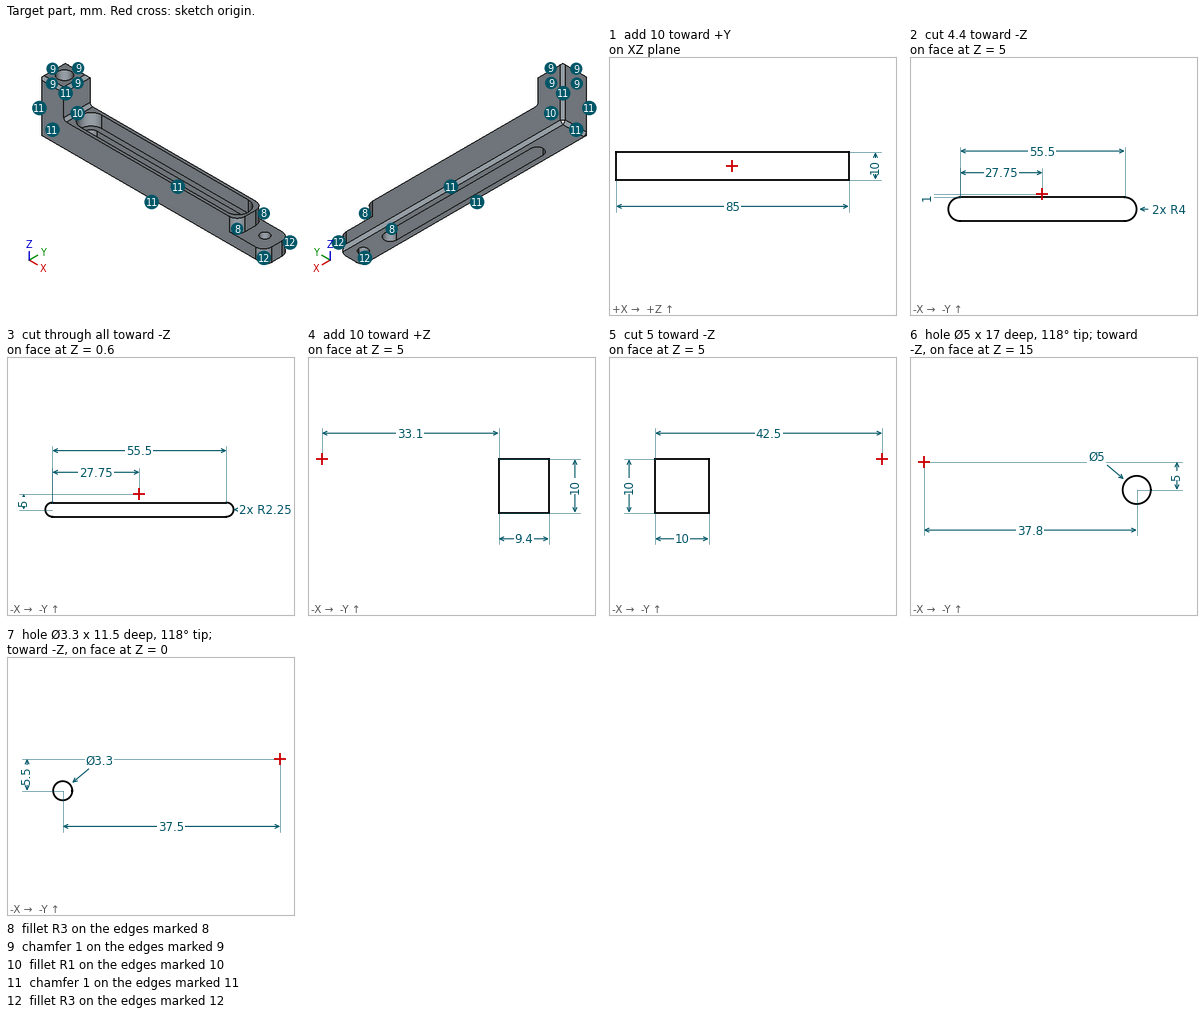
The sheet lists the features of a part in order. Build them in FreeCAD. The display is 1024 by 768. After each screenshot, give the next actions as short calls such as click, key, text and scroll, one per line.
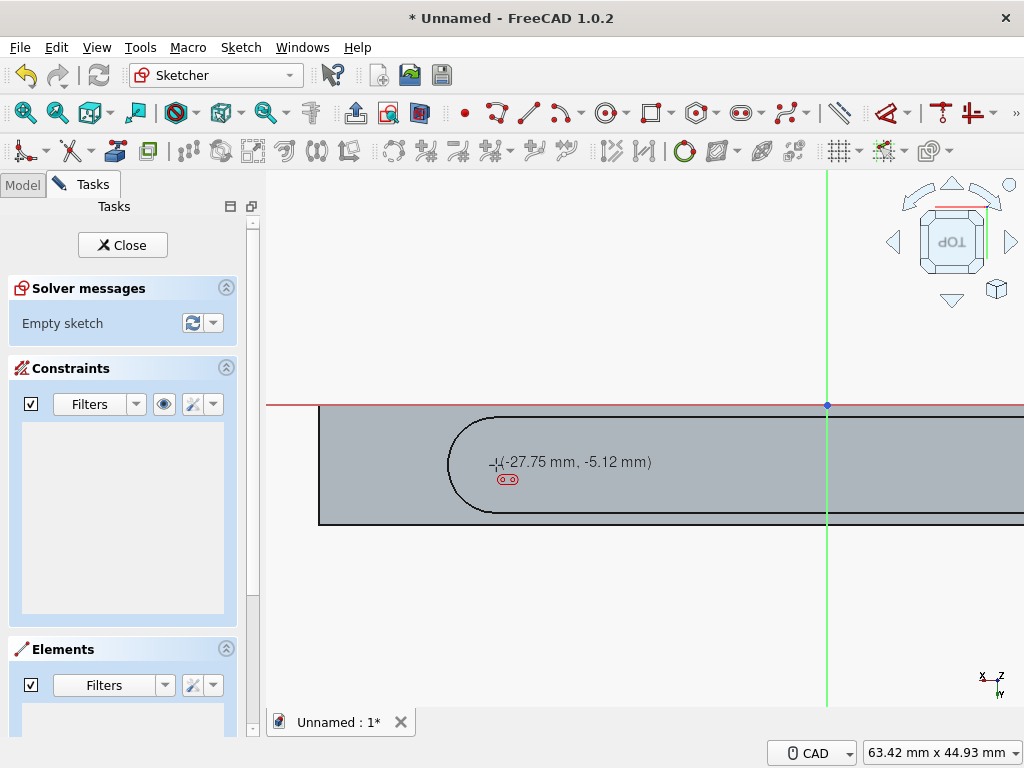
click(496, 465)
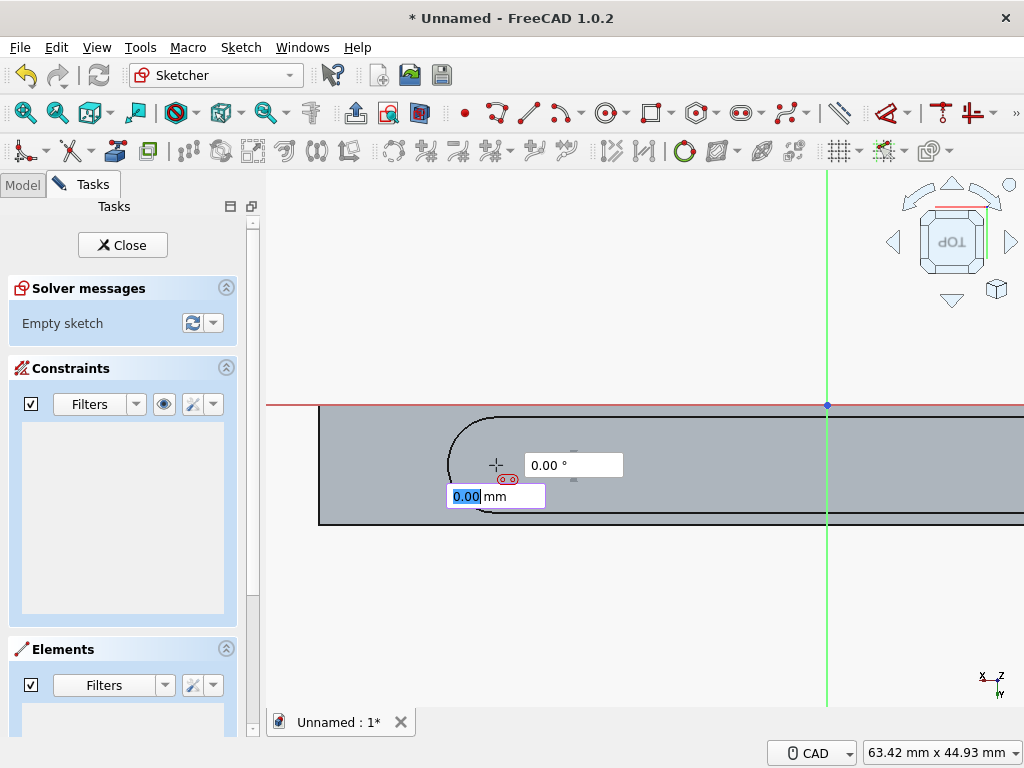
scroll(294, 426, down, 3)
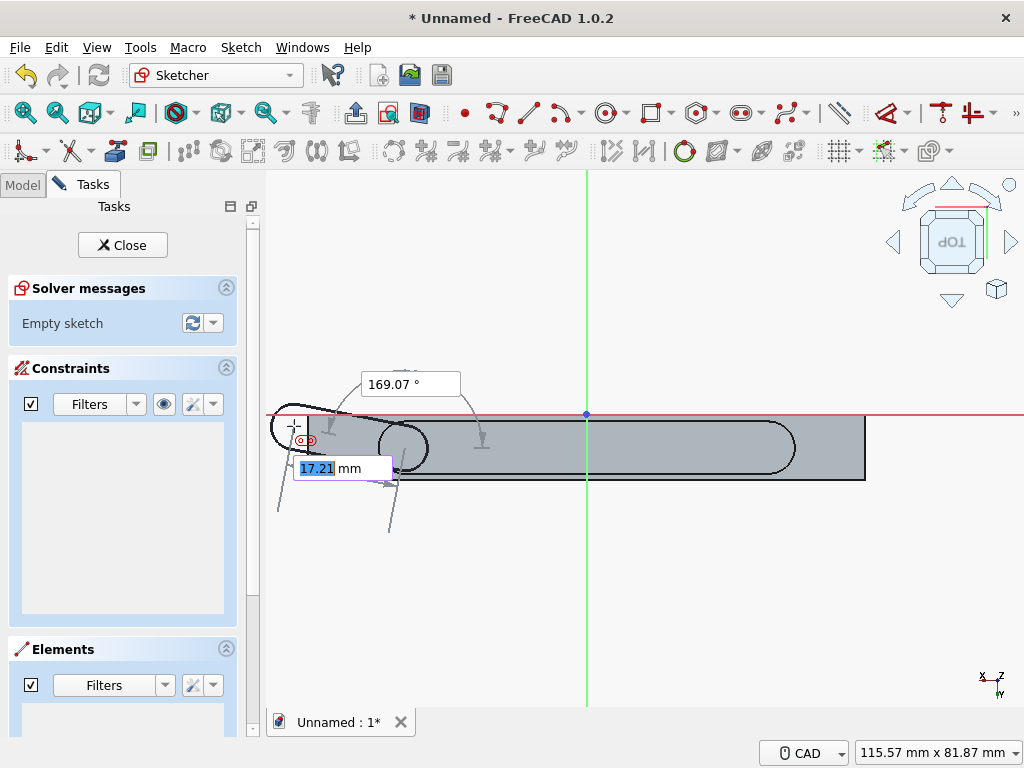
click(769, 448)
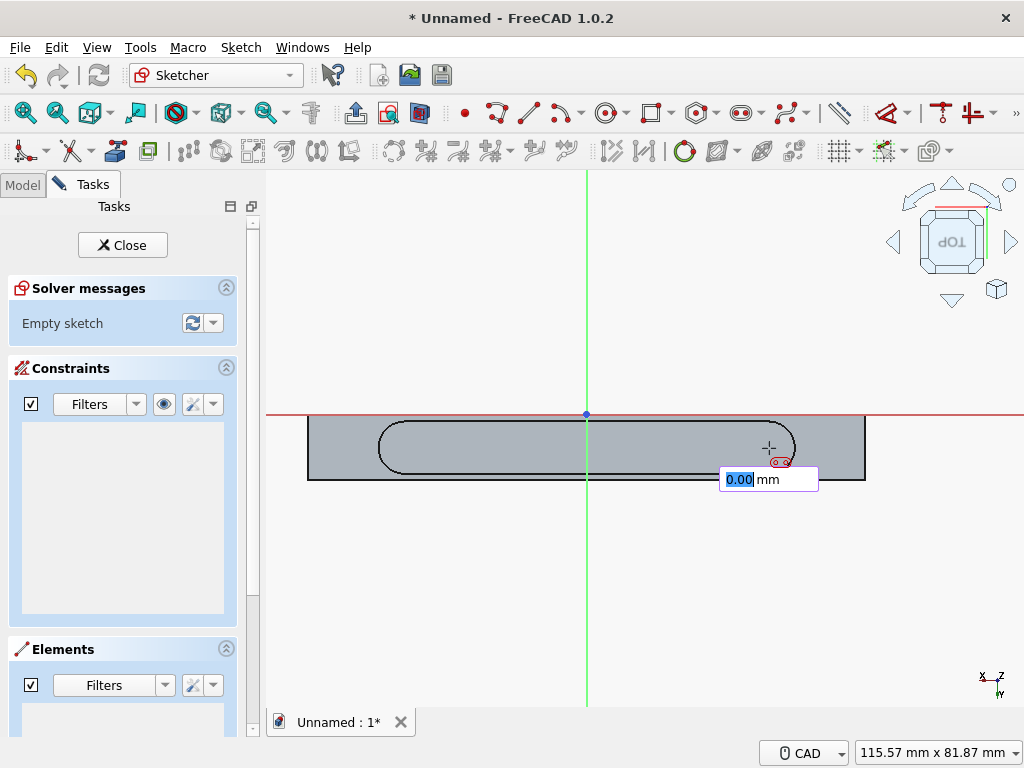
click(532, 462)
key(Escape)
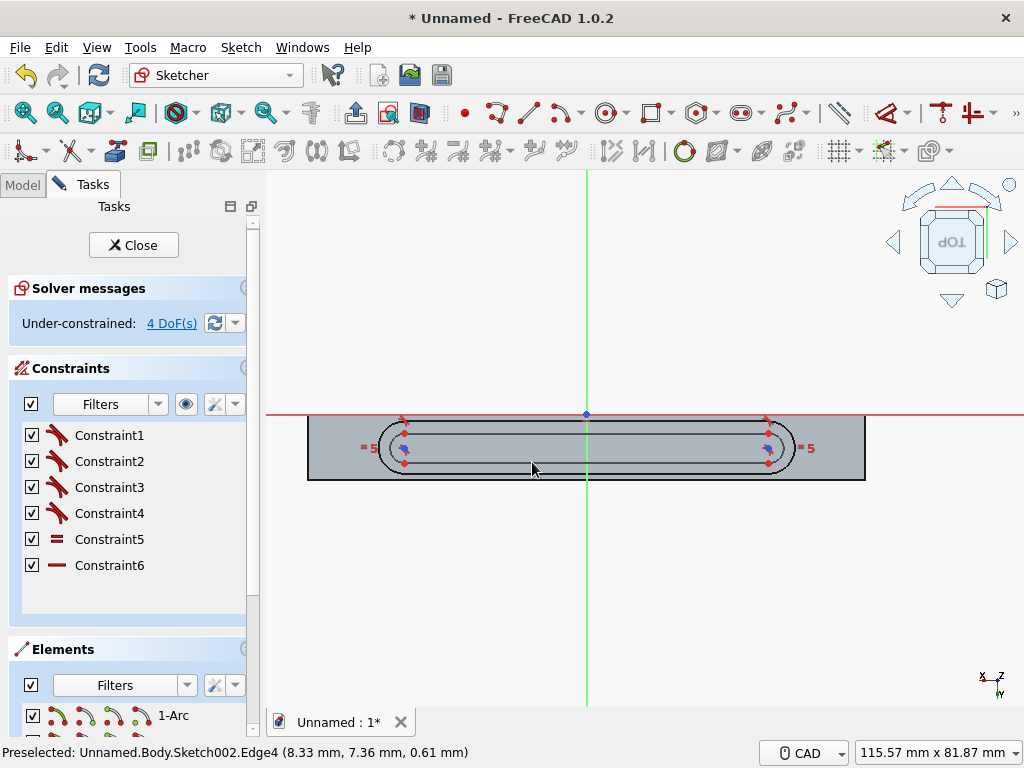
key(d)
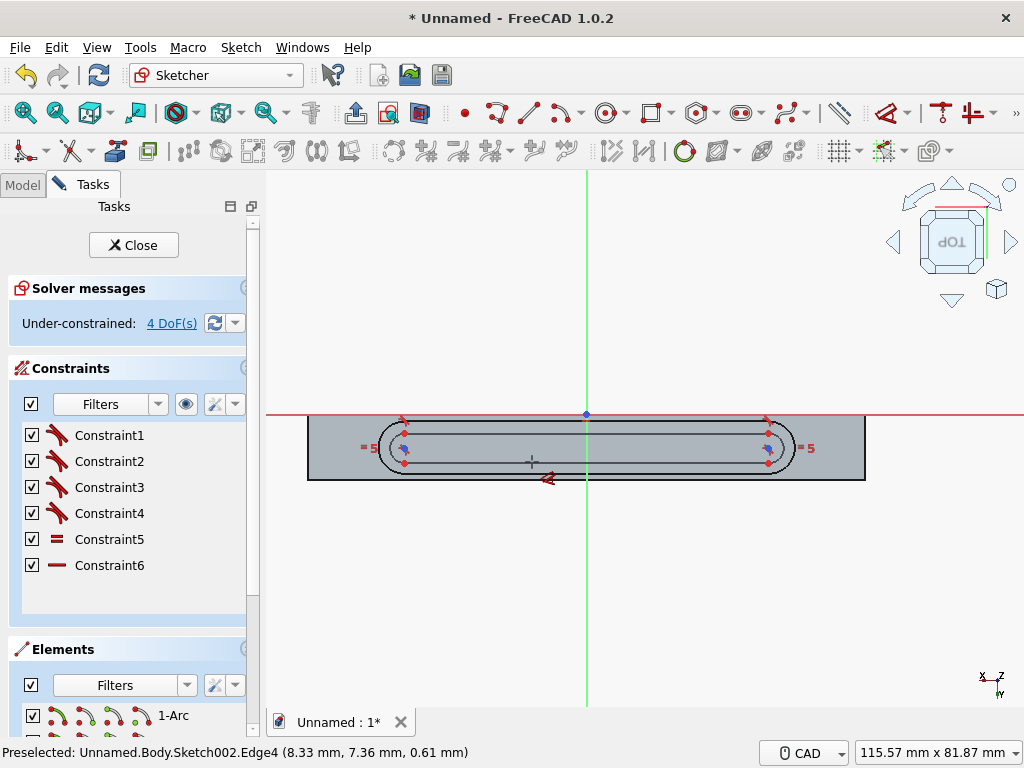
scroll(393, 440, up, 5)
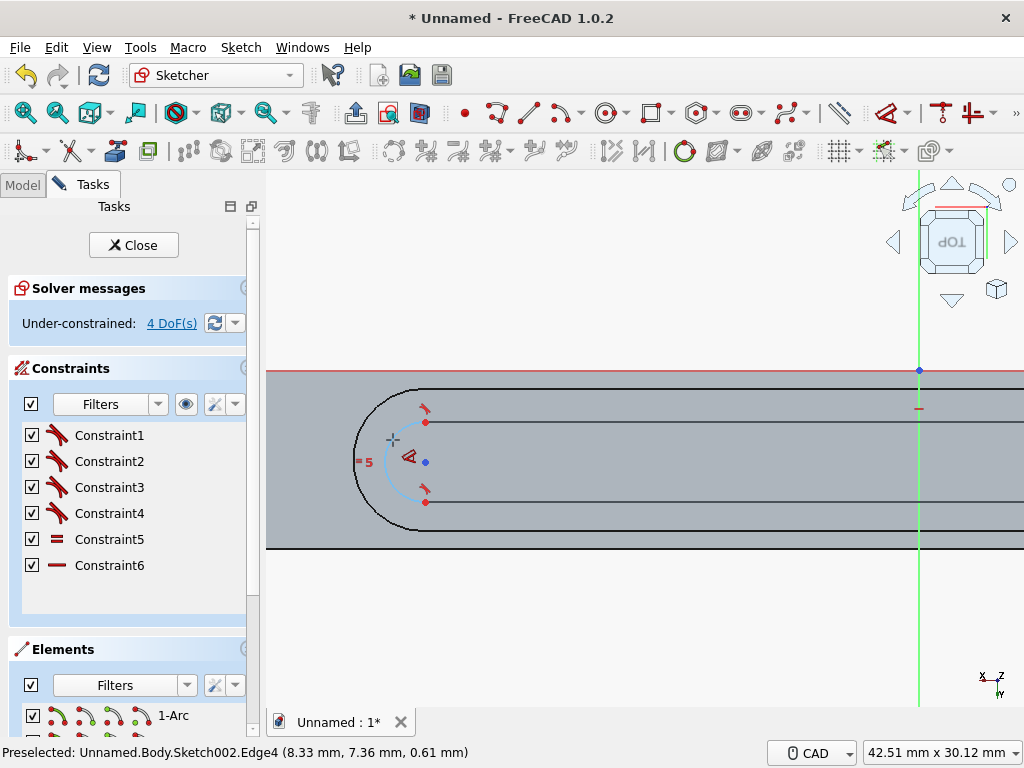
click(393, 439)
click(367, 420)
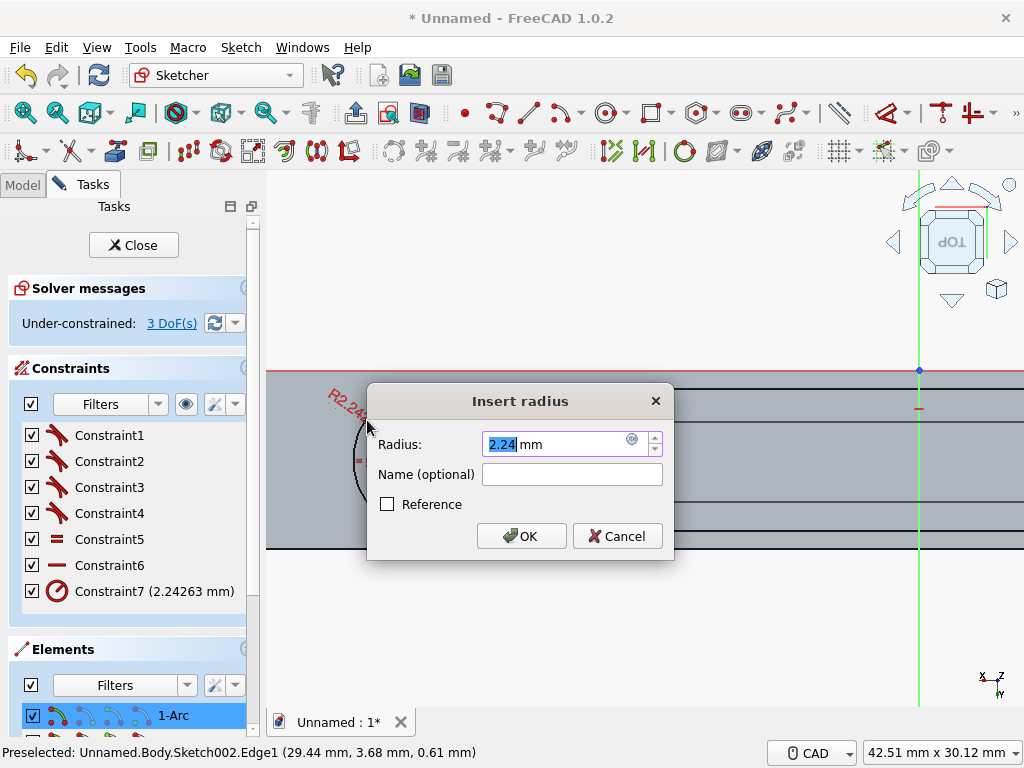
text(2.25)
key(Return)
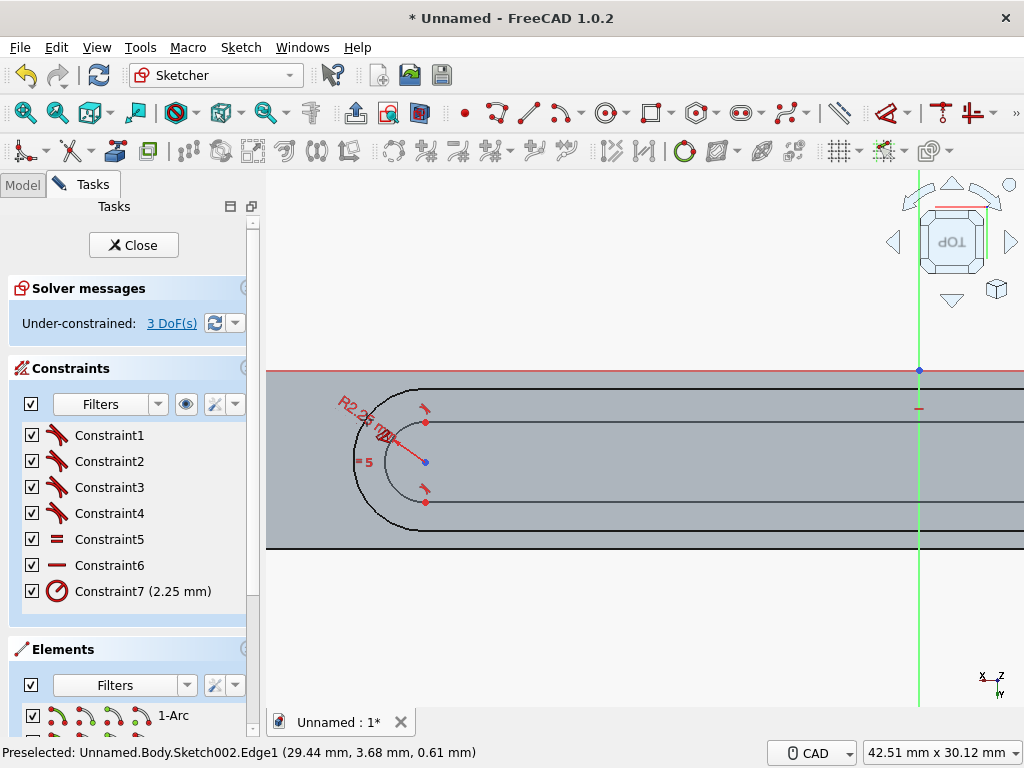
click(425, 462)
click(391, 396)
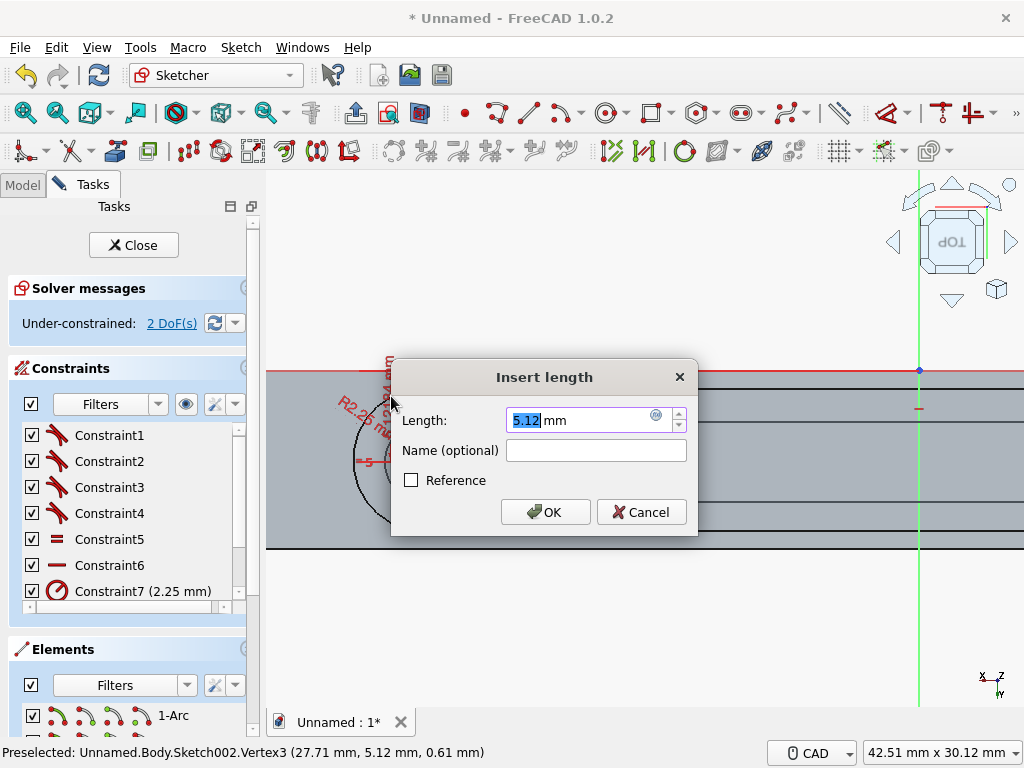
text(5)
key(Return)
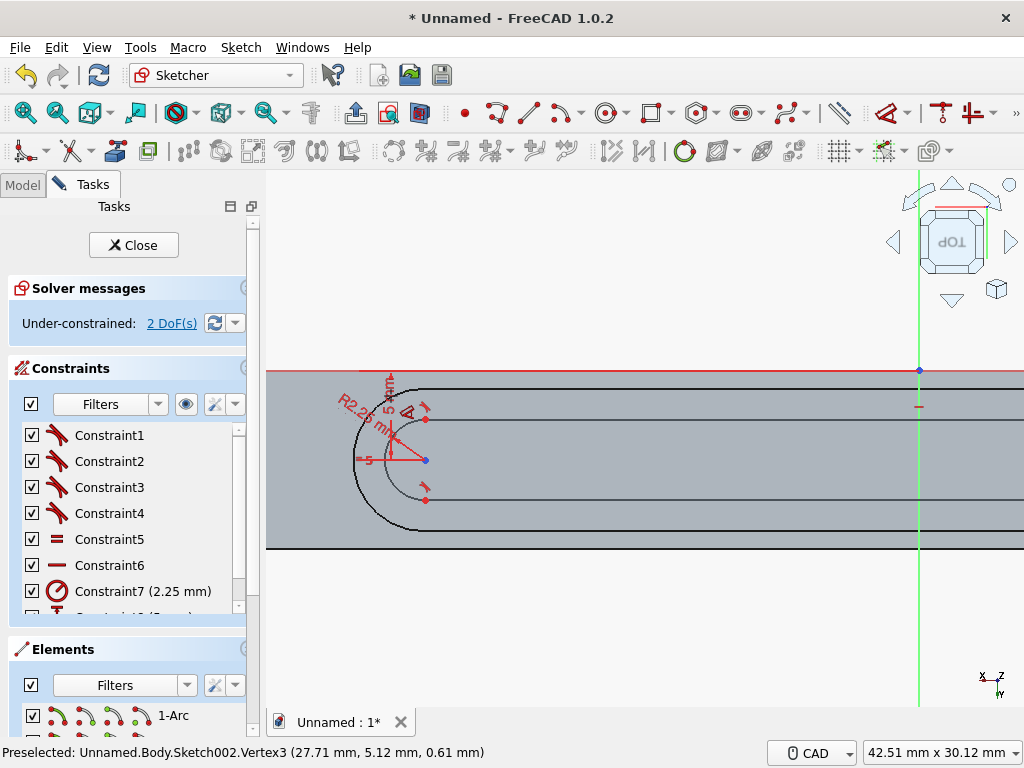
click(722, 420)
click(642, 386)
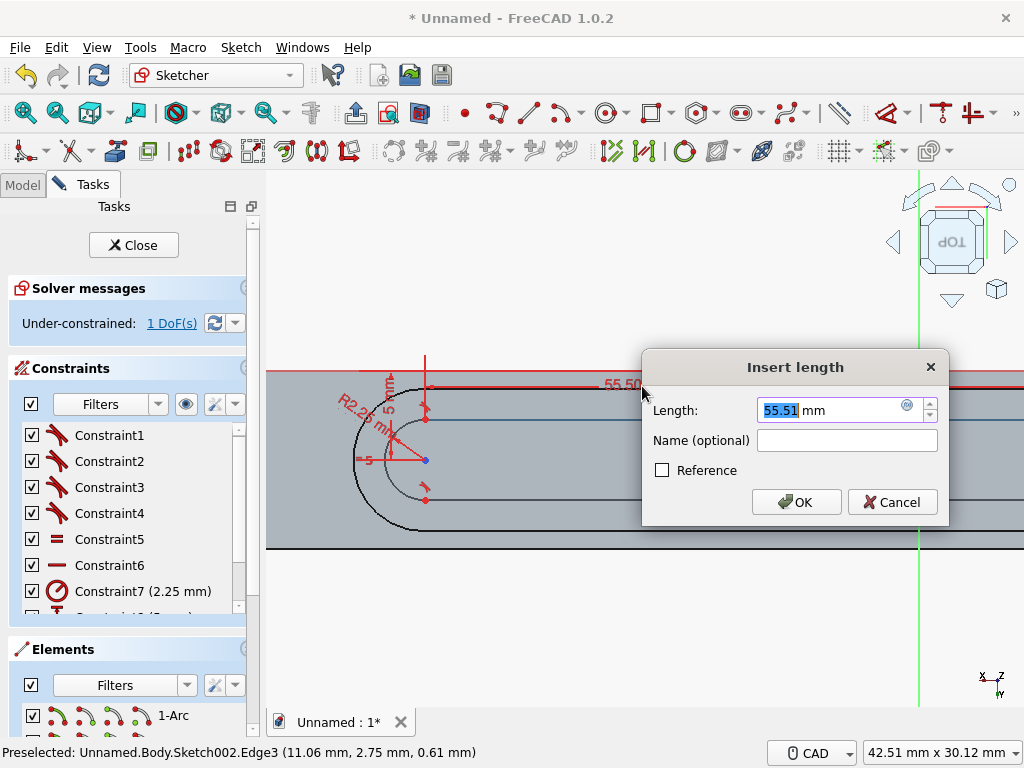
text(55.5)
key(Return)